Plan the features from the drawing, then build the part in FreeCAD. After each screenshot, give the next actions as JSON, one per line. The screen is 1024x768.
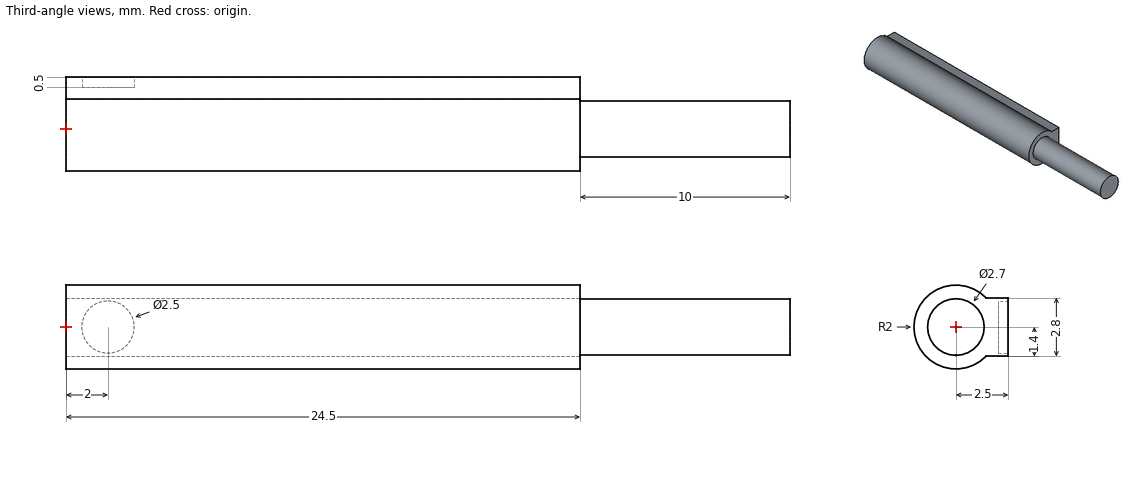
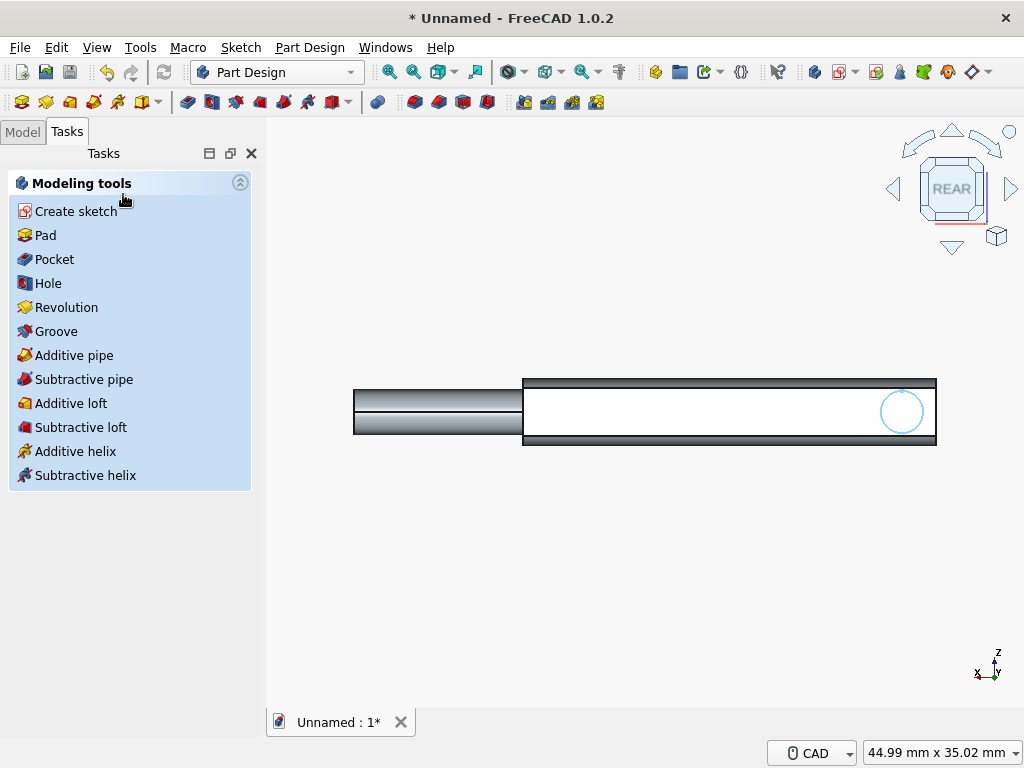
{"action": "left_click", "coordinate": [188, 102]}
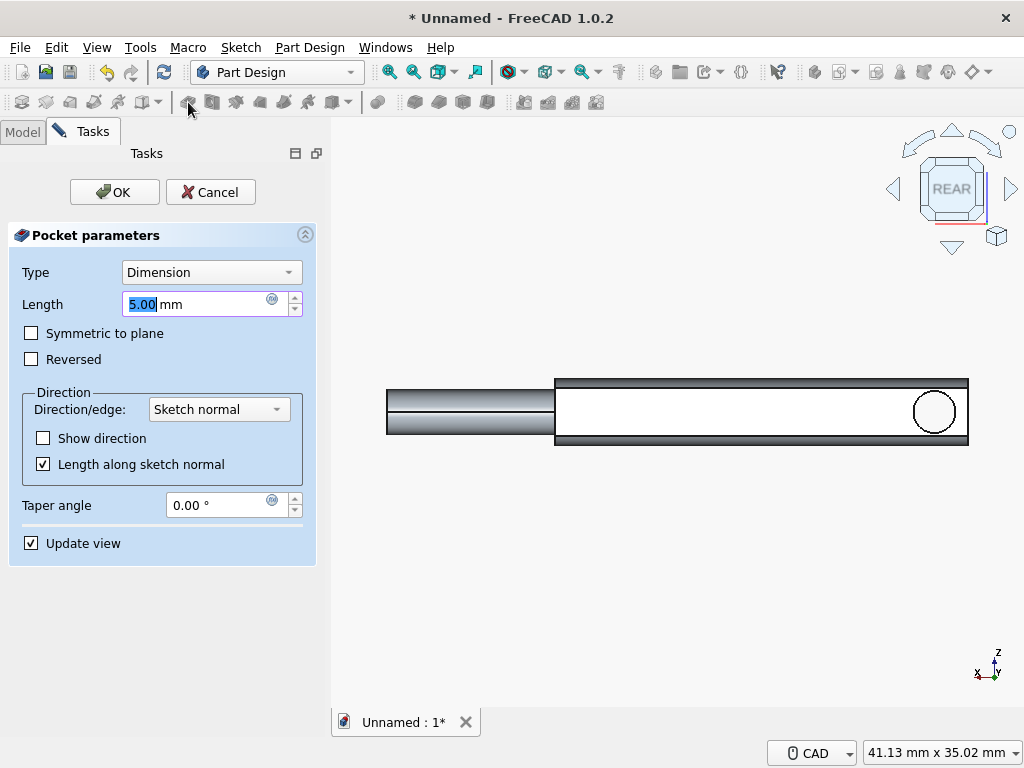
{"action": "type", "text": "0.5"}
{"action": "key", "text": "Tab"}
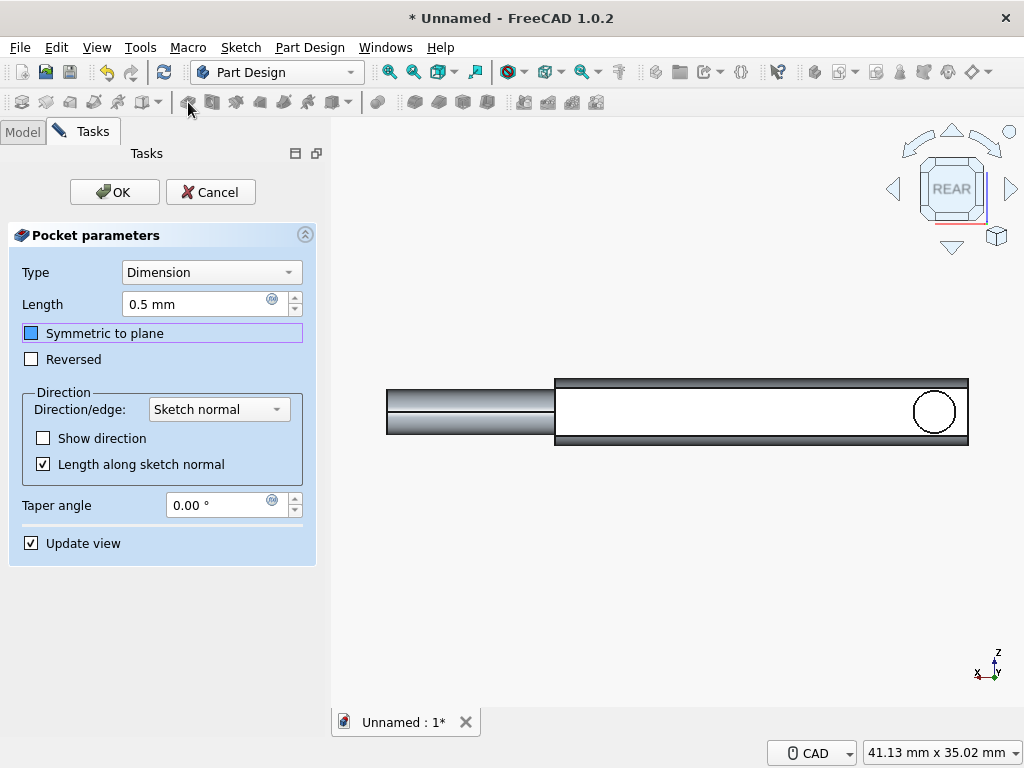
{"action": "left_click", "coordinate": [115, 192]}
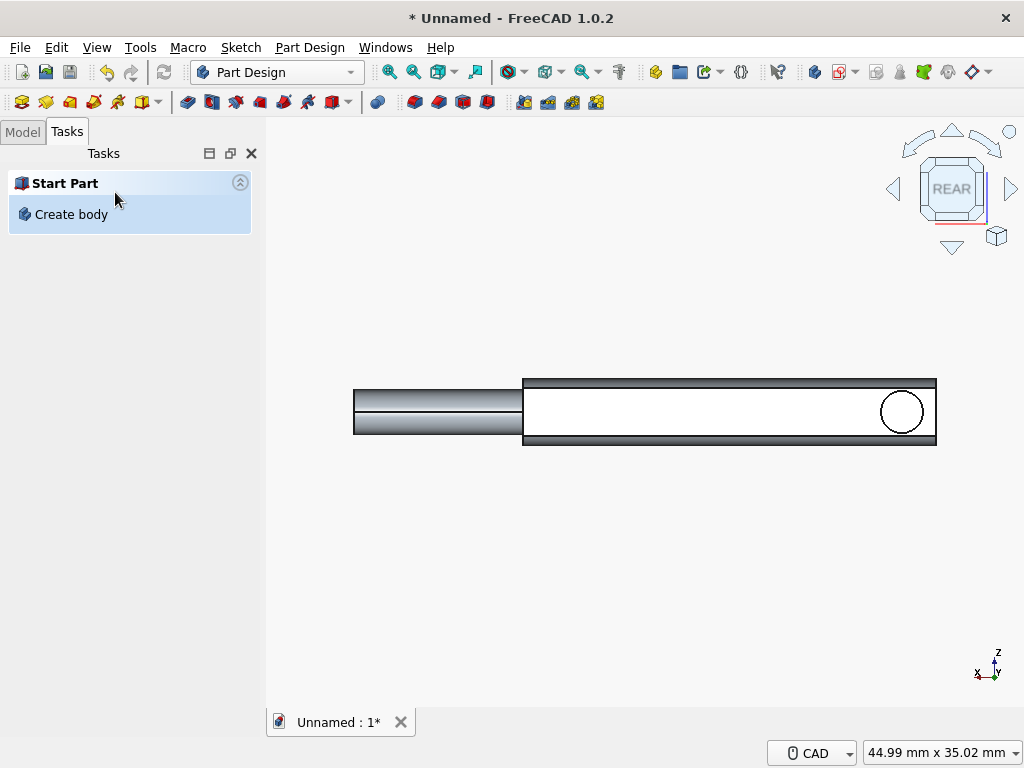
{"action": "key", "text": "0"}